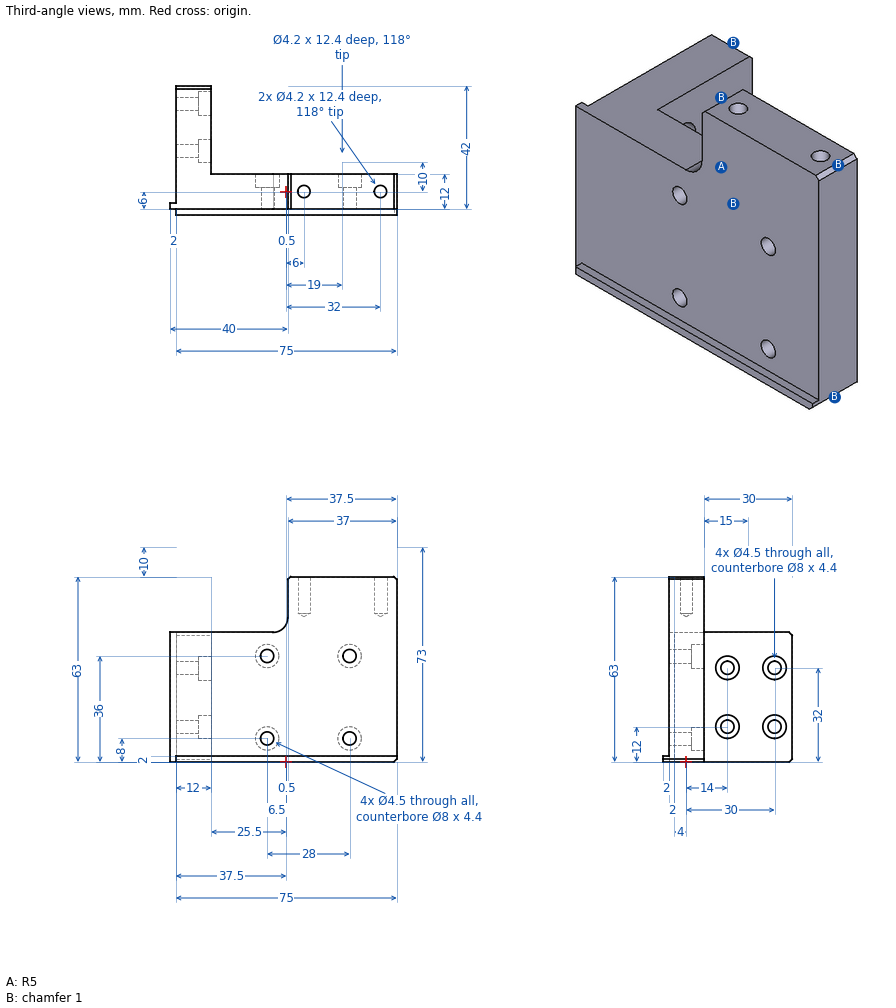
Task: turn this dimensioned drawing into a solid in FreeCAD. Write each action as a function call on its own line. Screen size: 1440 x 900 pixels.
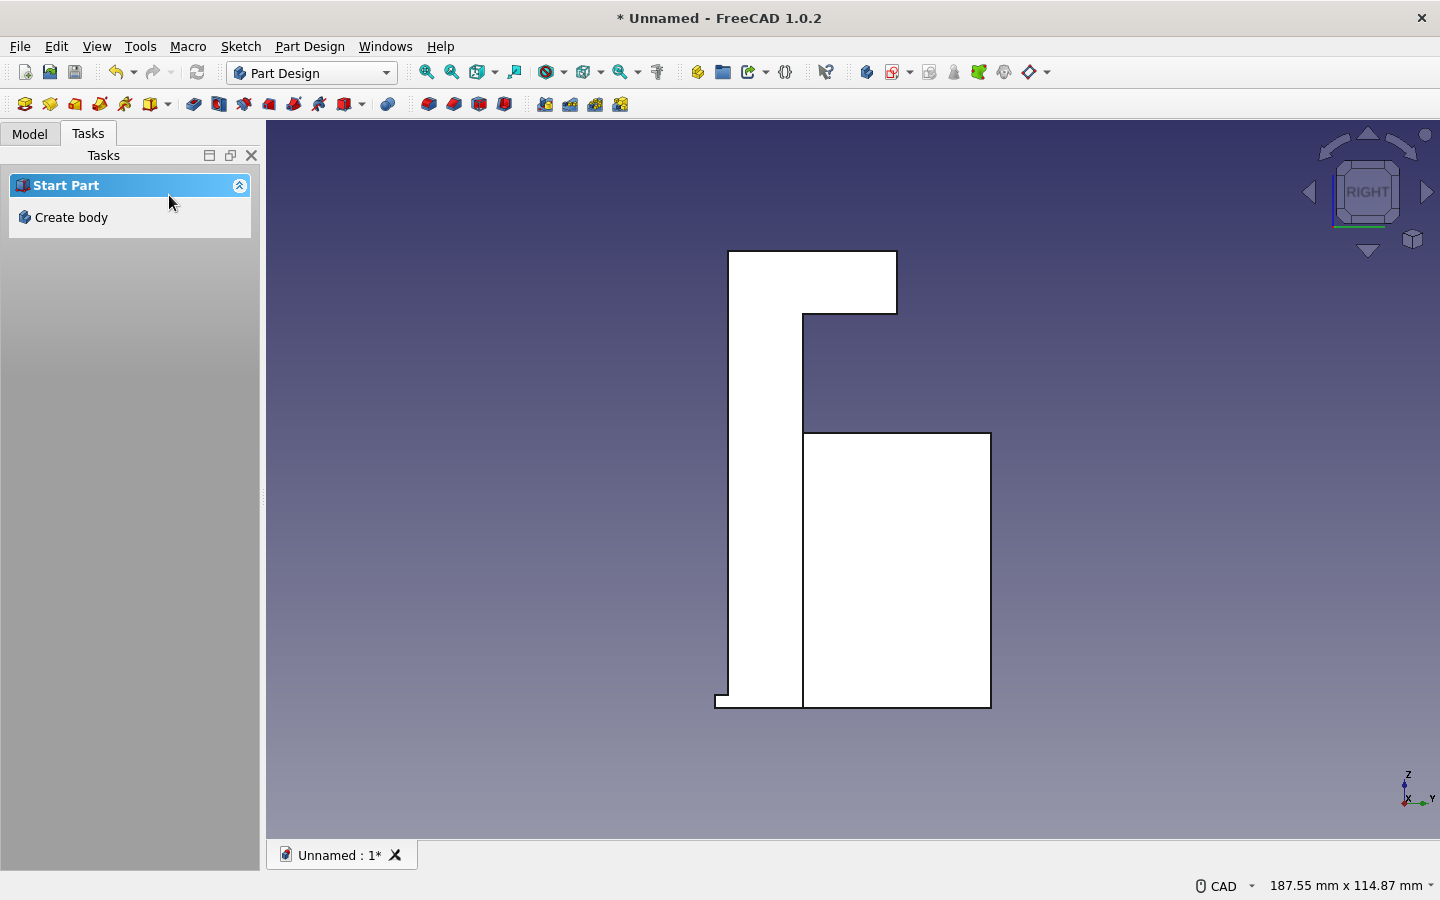
click(897, 530)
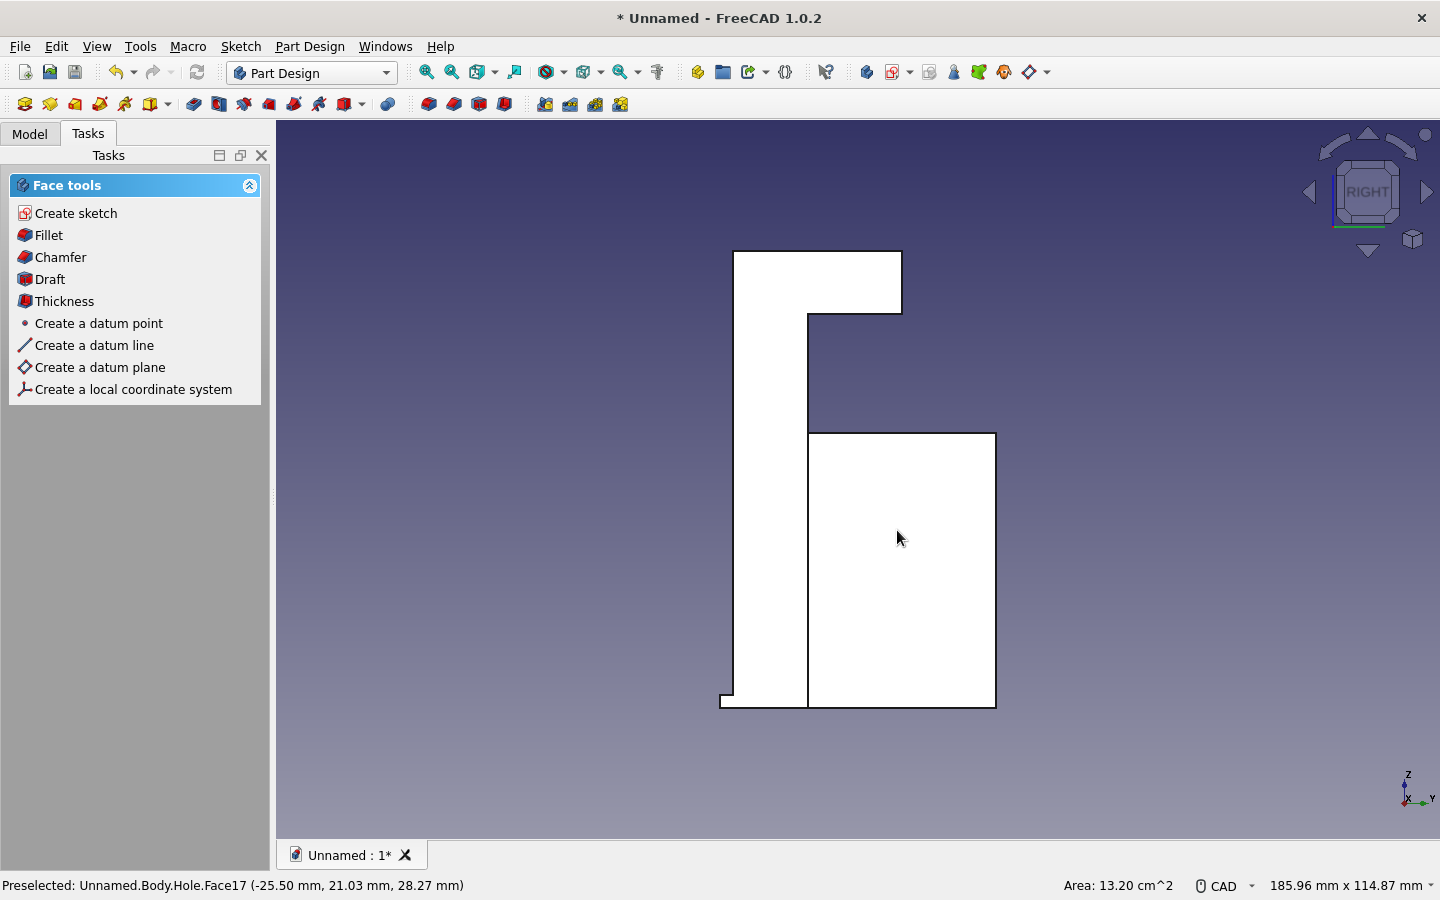
click(892, 72)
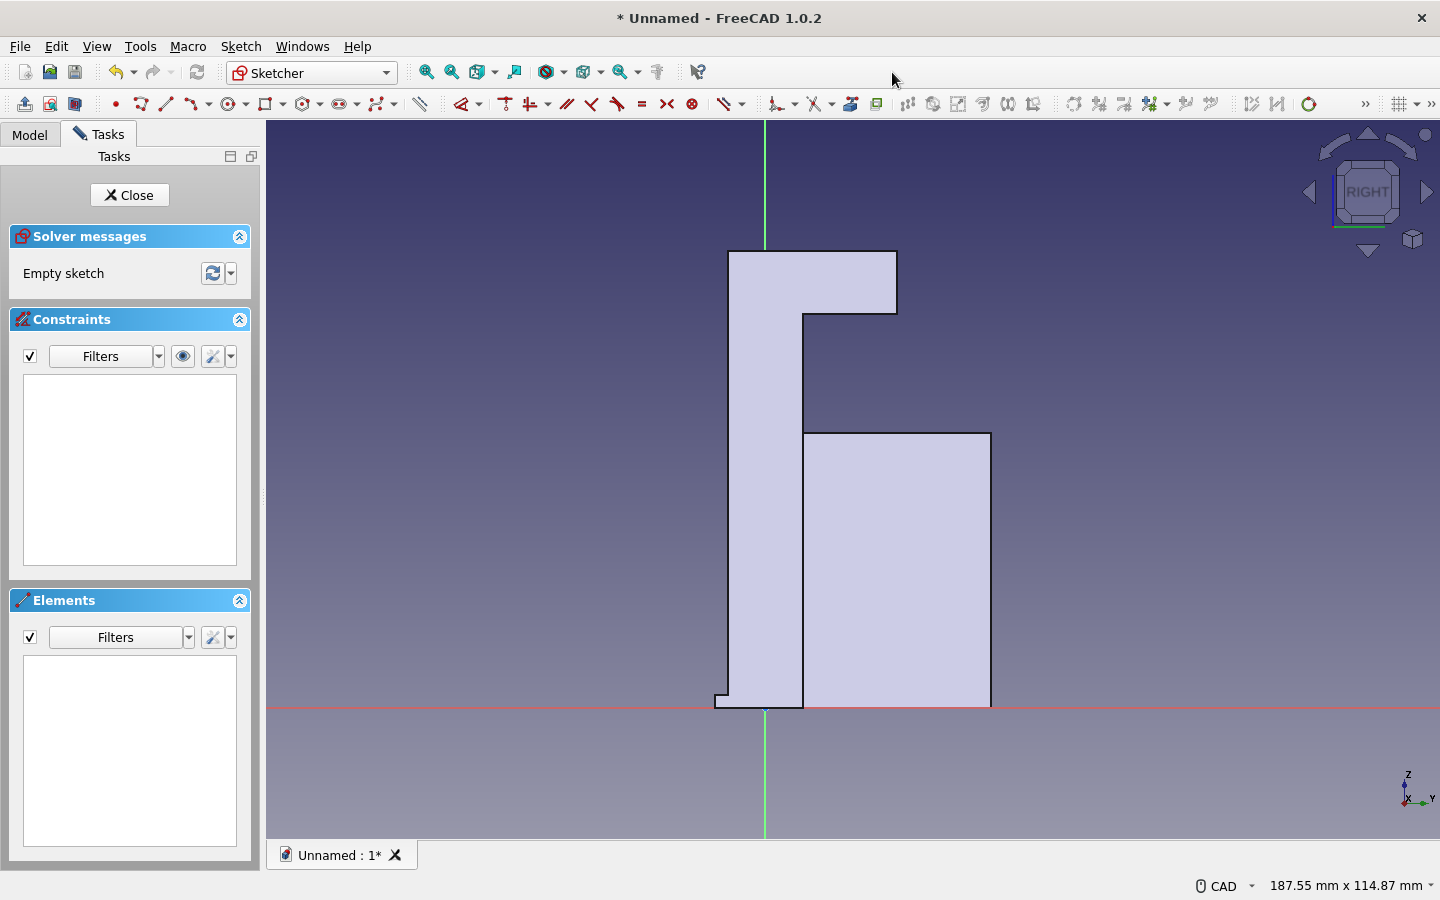
scroll(933, 700, up, 4)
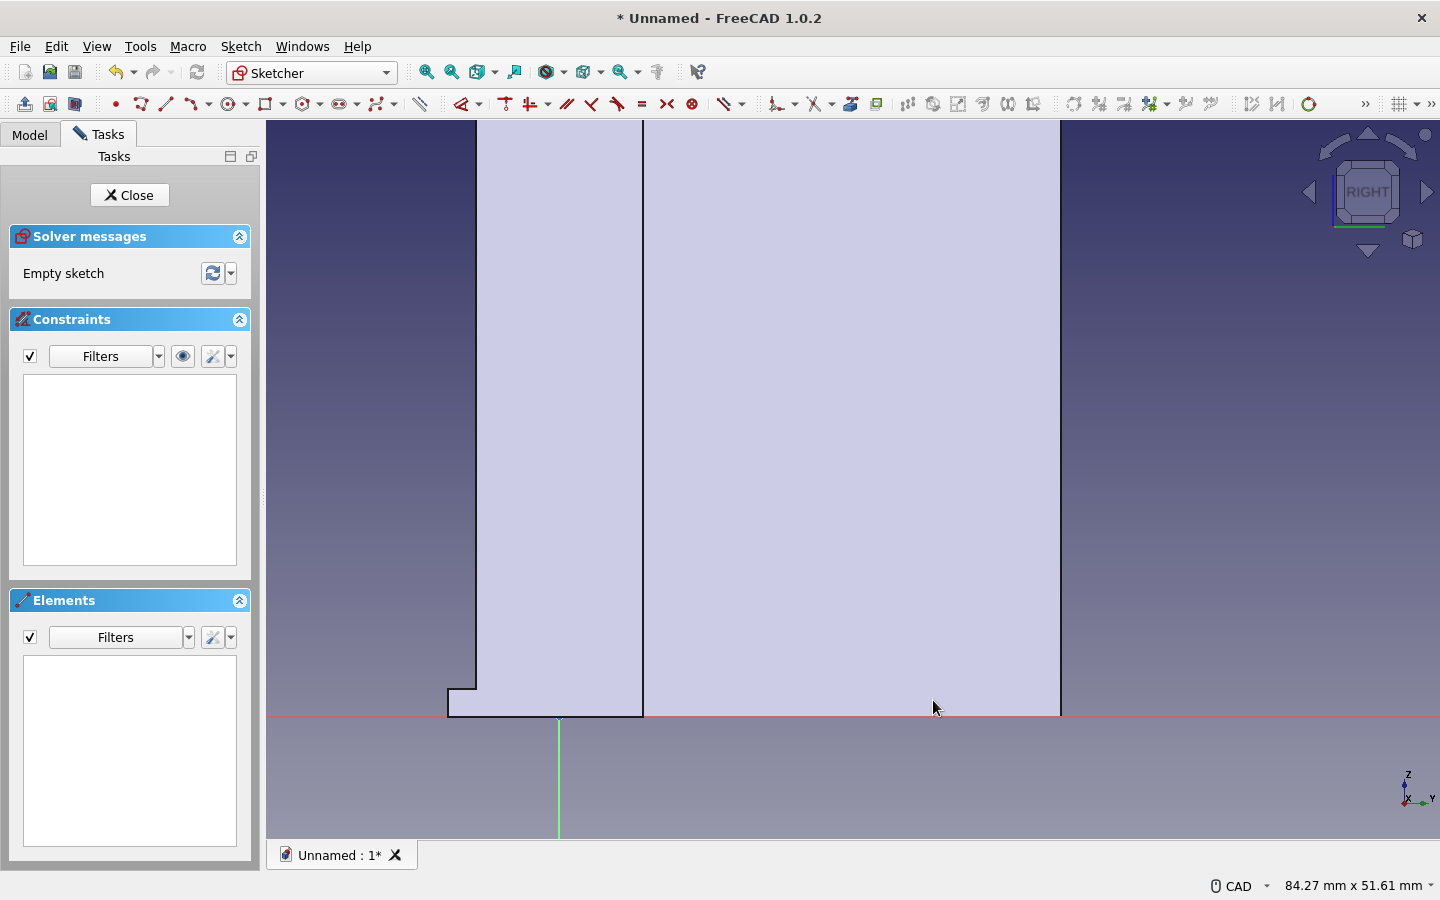
click(228, 104)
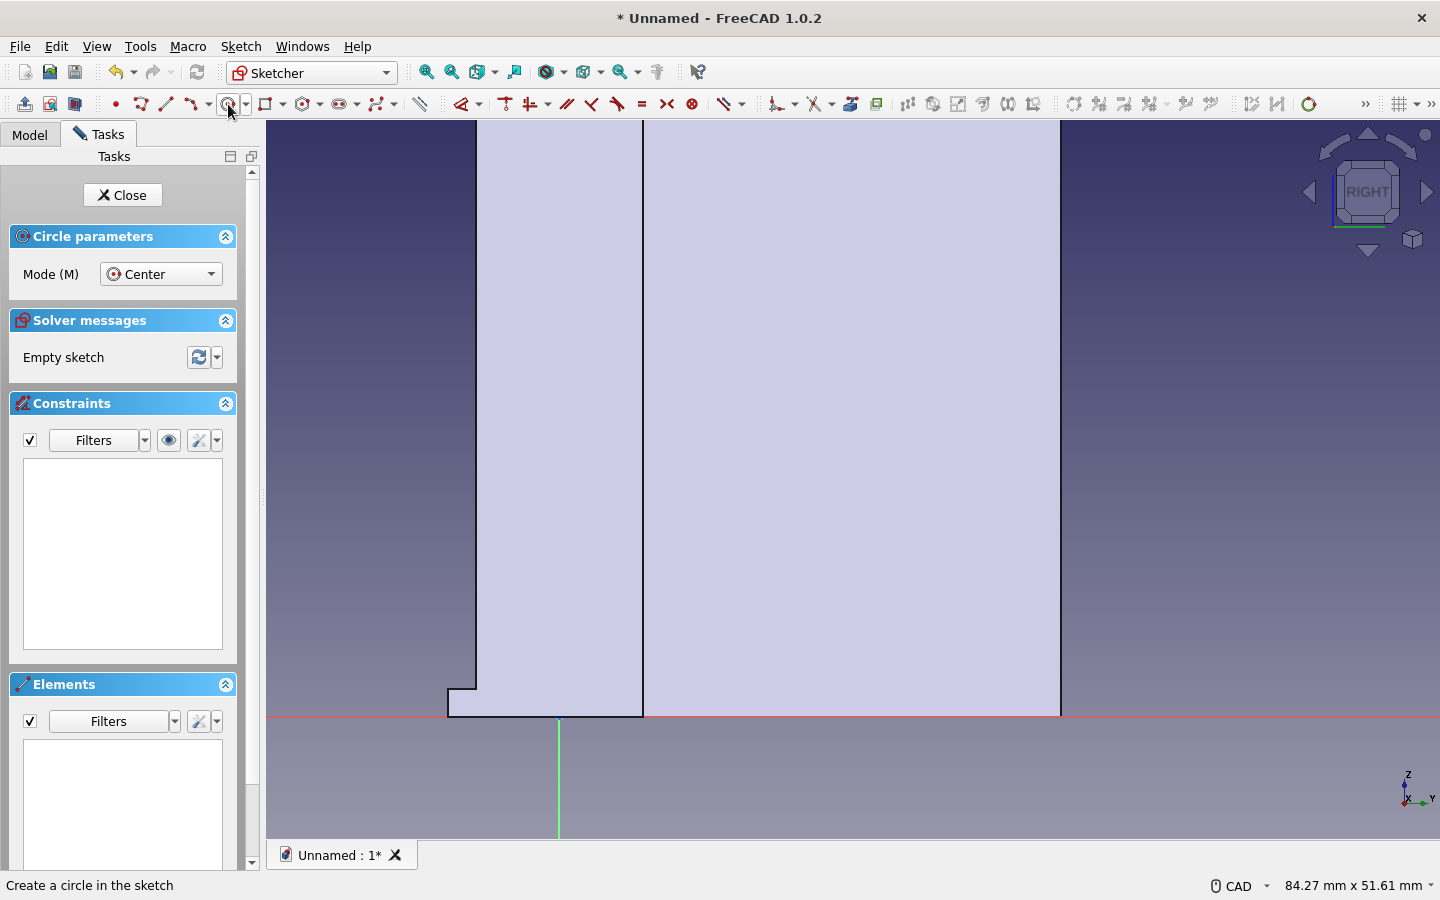
click(977, 271)
move(999, 249)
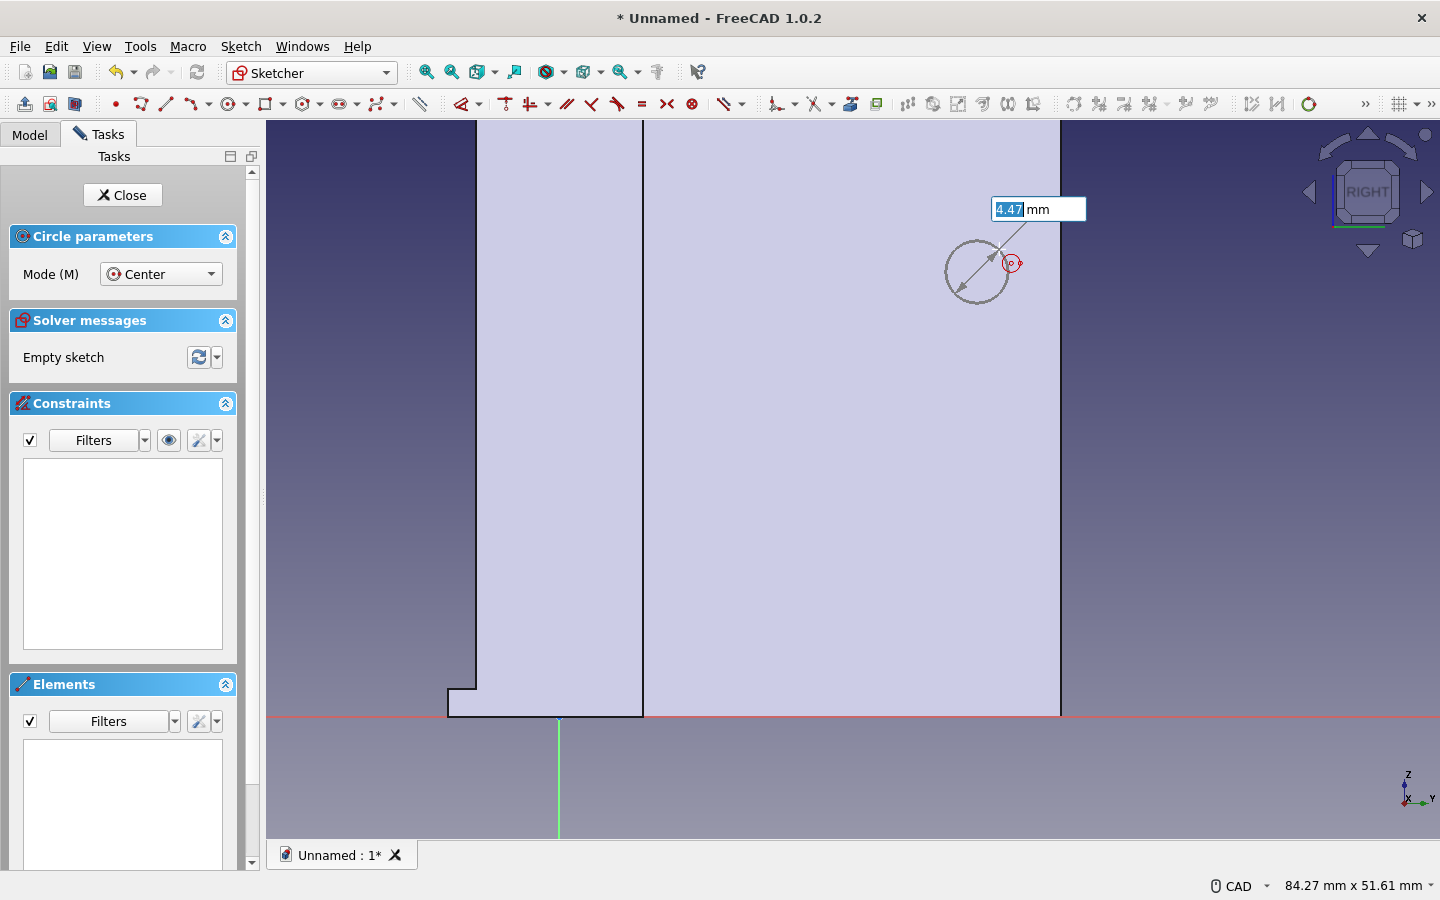
text(4.5)
key(Return)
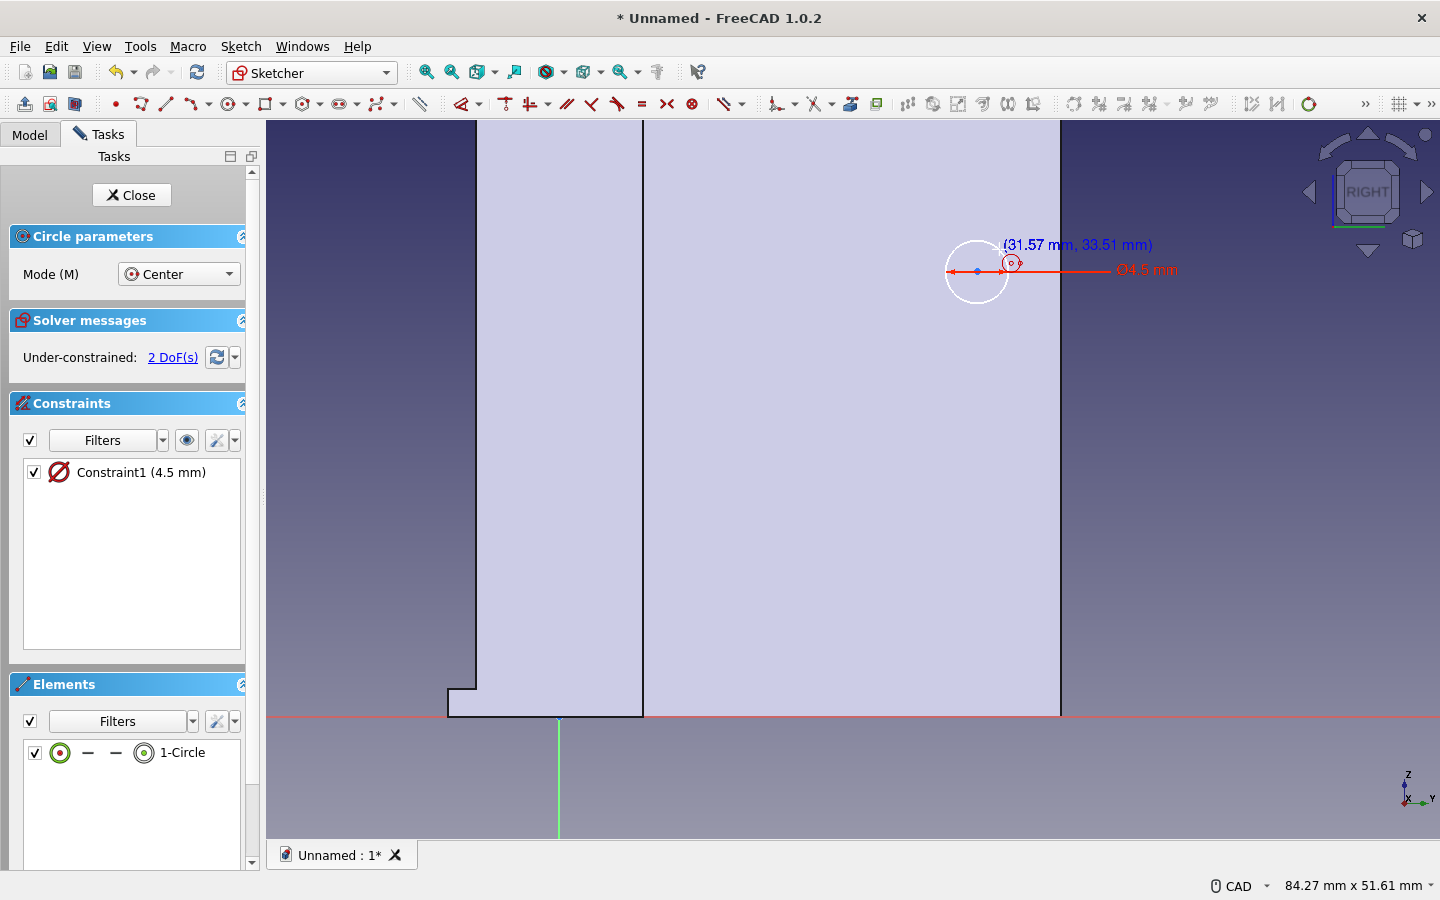
click(754, 271)
move(776, 249)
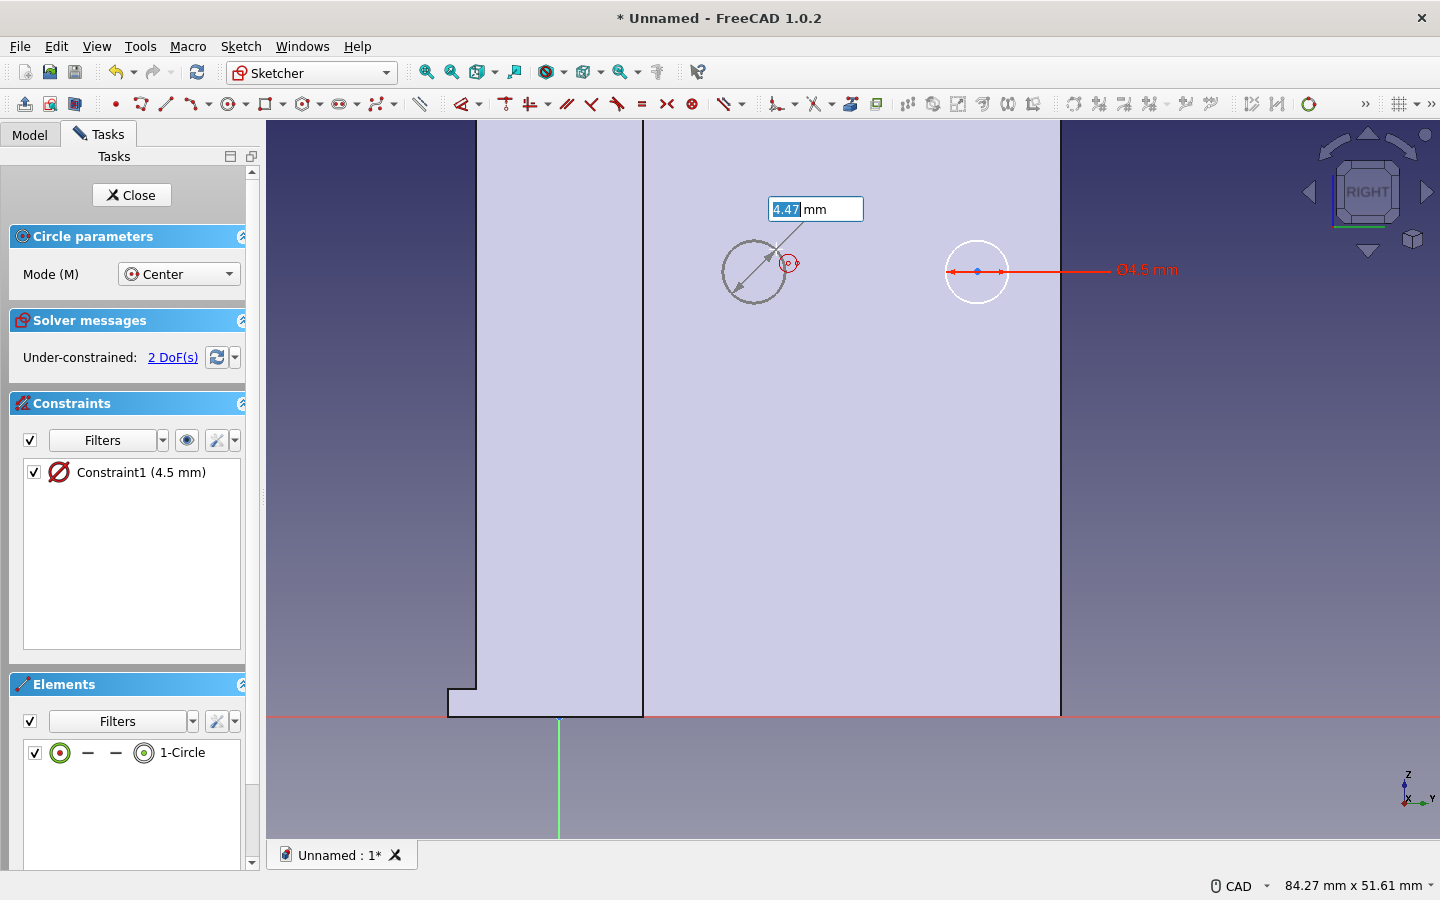
text(4.5)
key(Return)